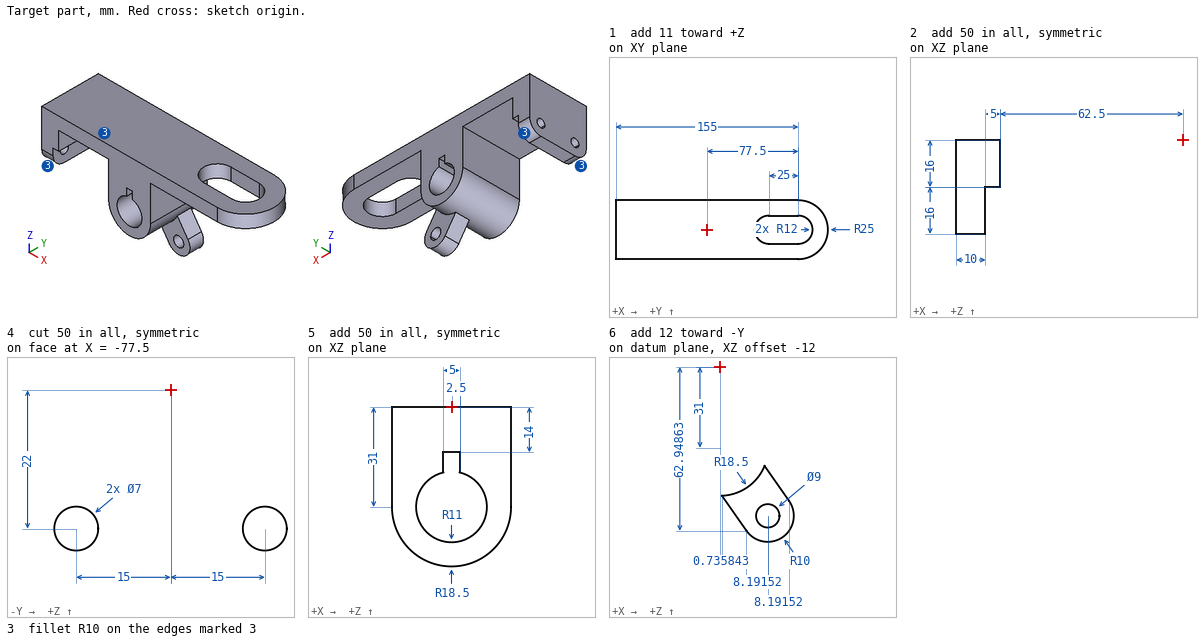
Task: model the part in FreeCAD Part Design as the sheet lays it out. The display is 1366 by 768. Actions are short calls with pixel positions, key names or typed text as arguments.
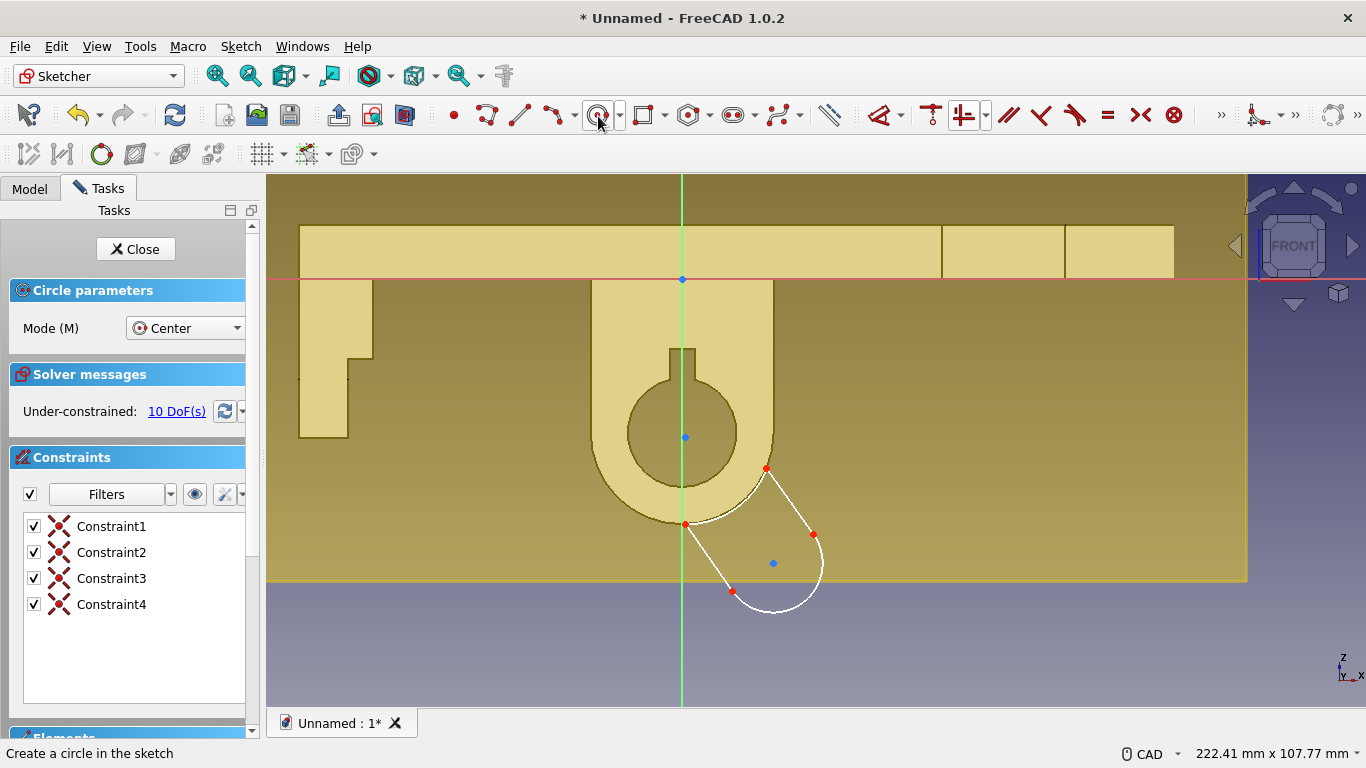
click(773, 562)
click(789, 547)
key(Escape)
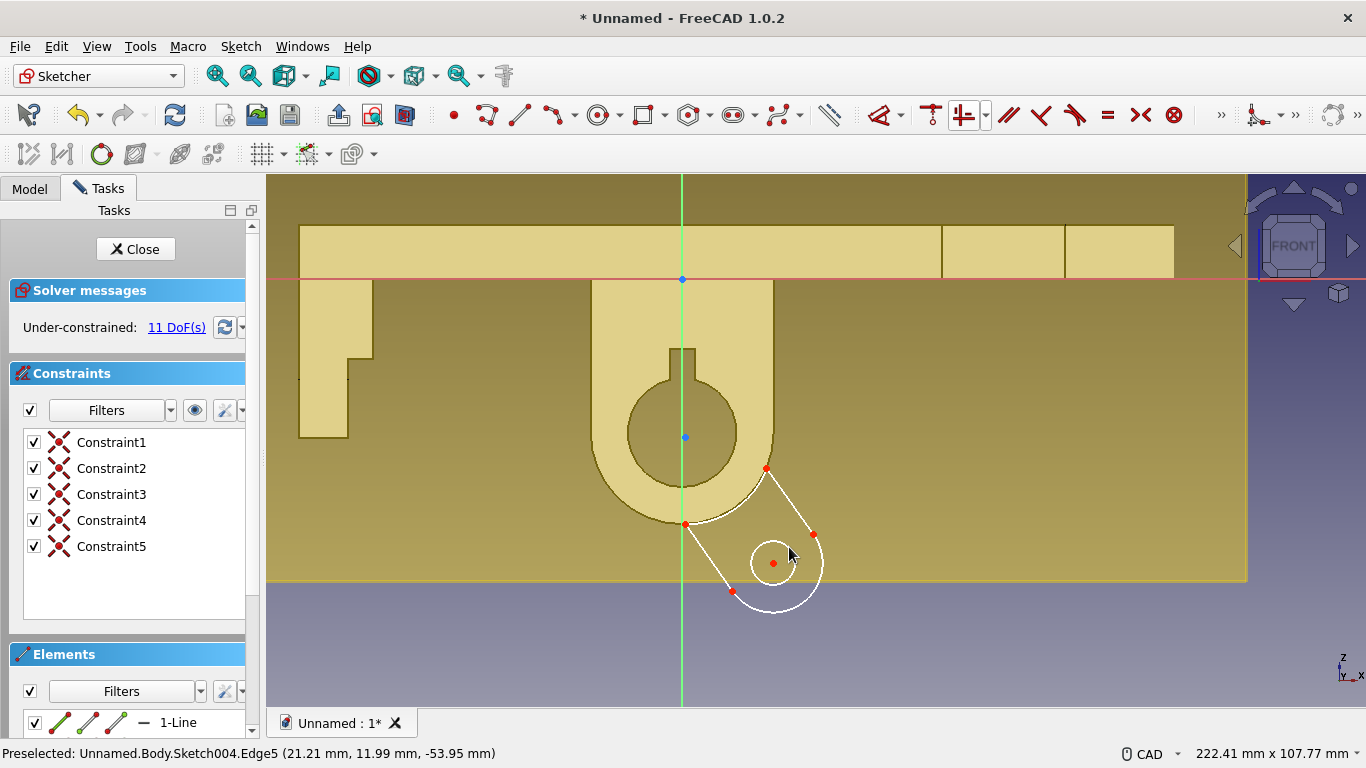
click(781, 489)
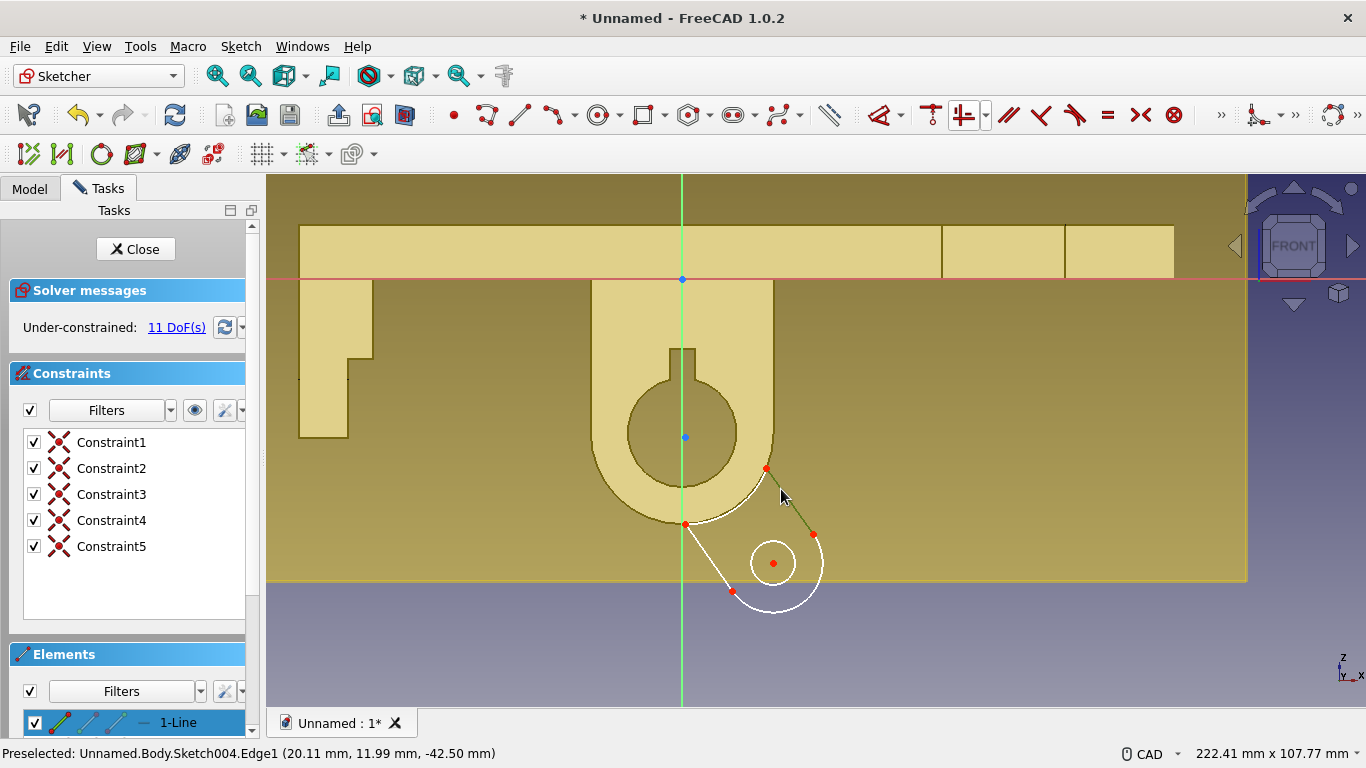
click(772, 613)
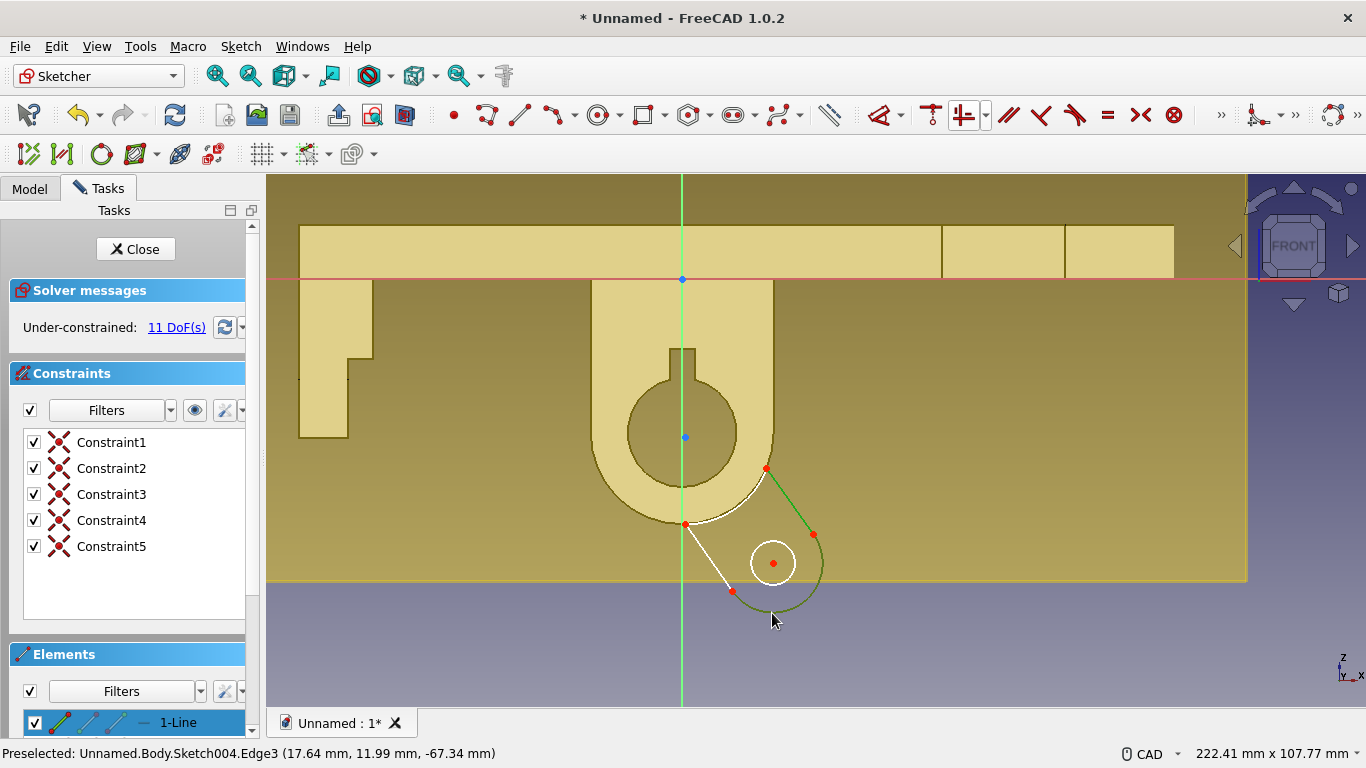
click(1075, 116)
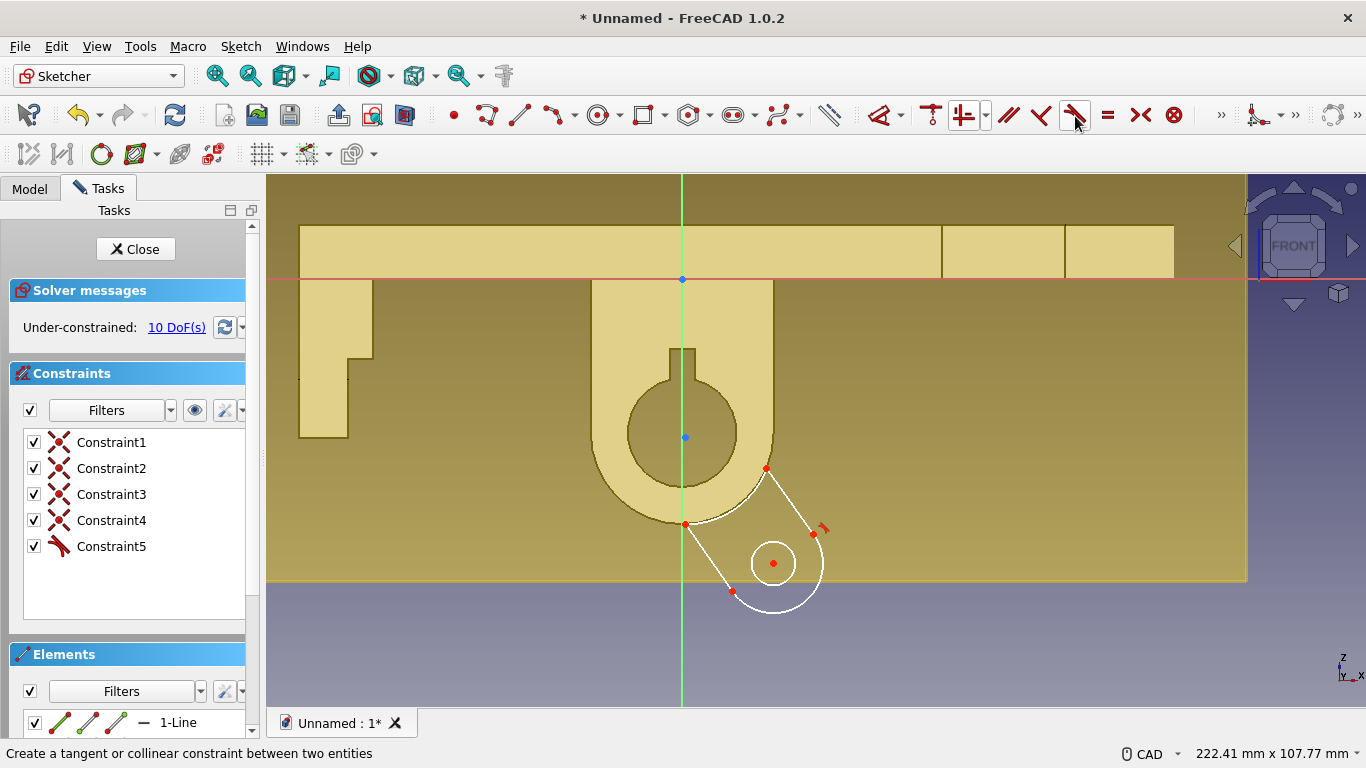
click(719, 572)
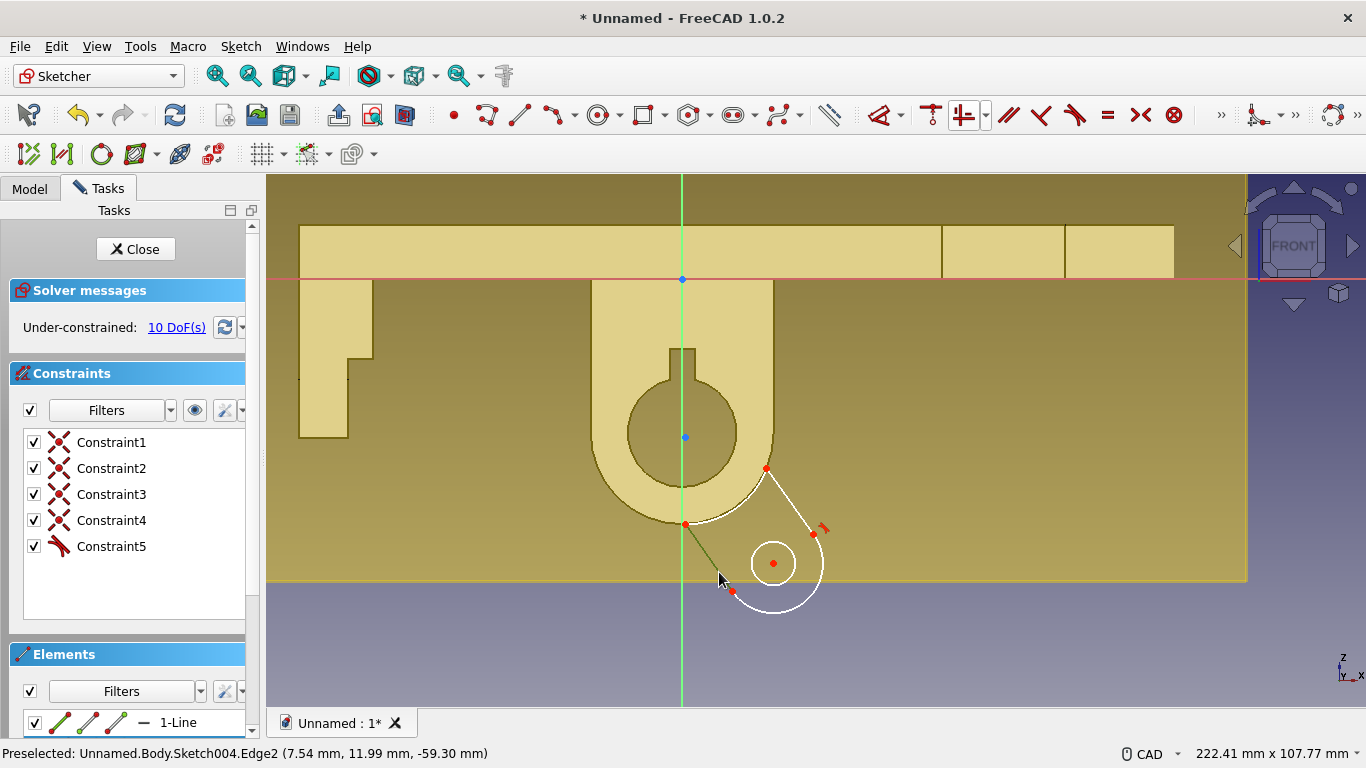
click(773, 613)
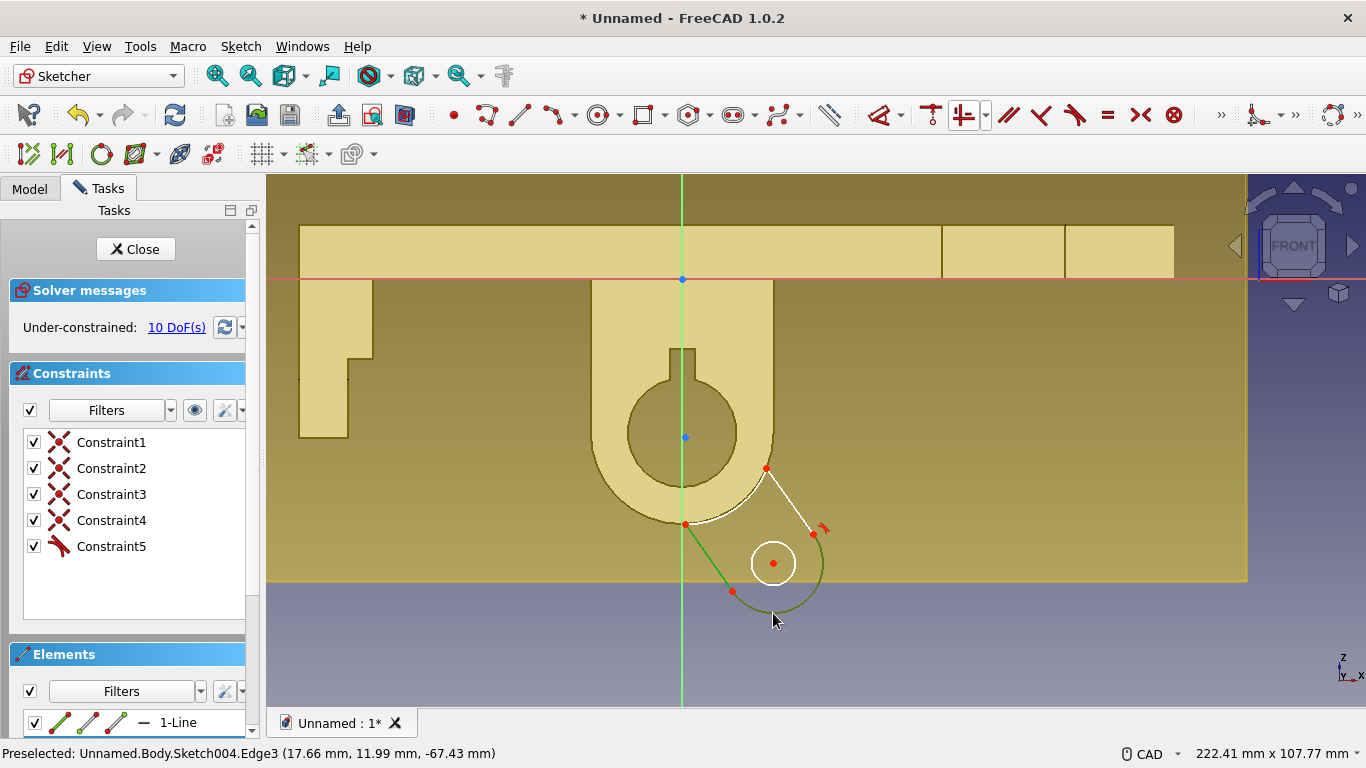
click(1075, 116)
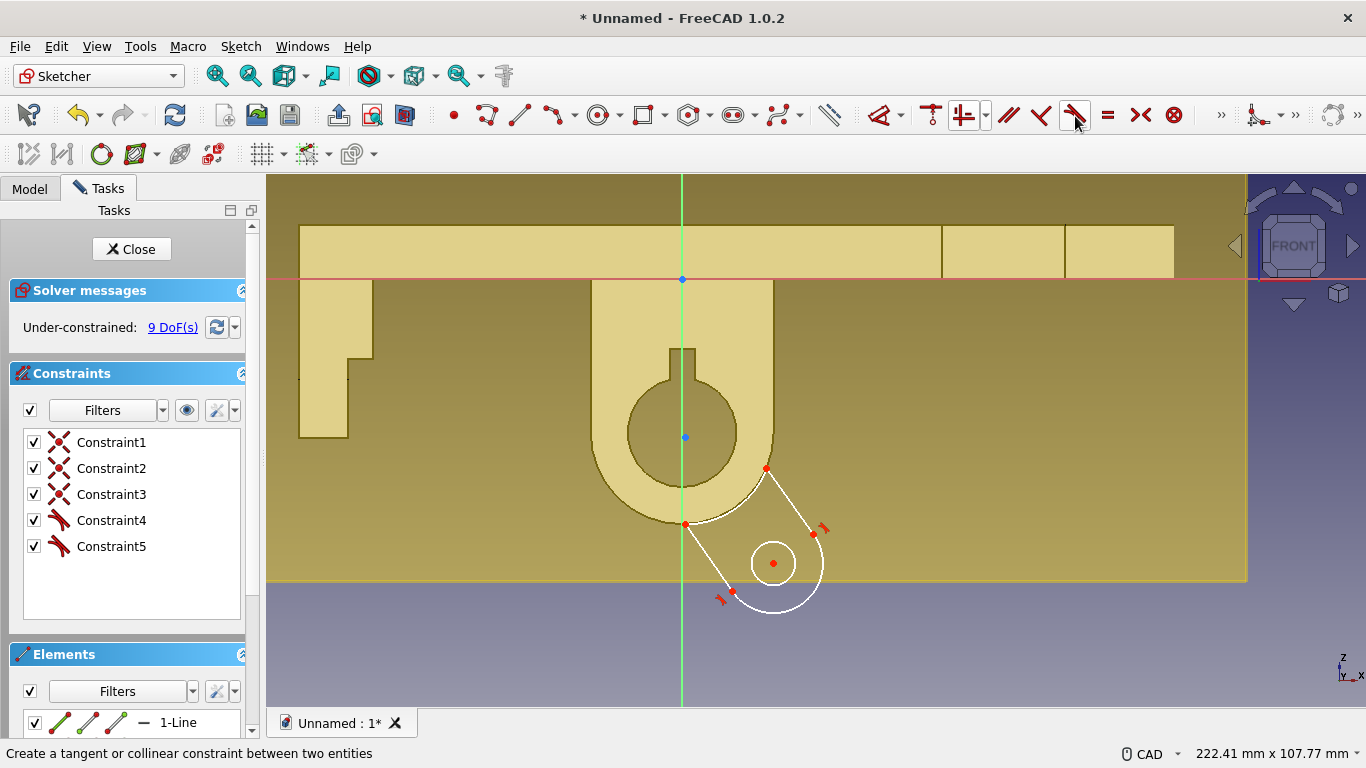
click(686, 437)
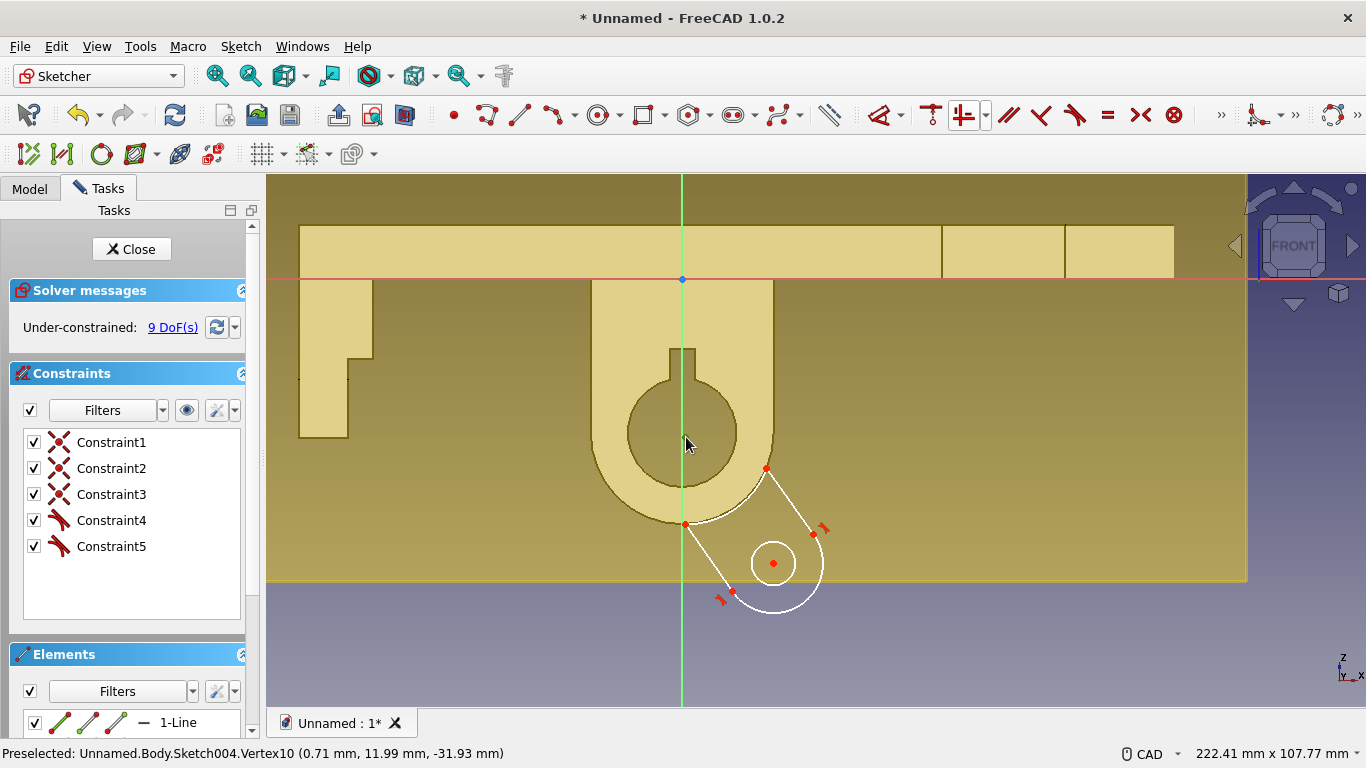
click(682, 645)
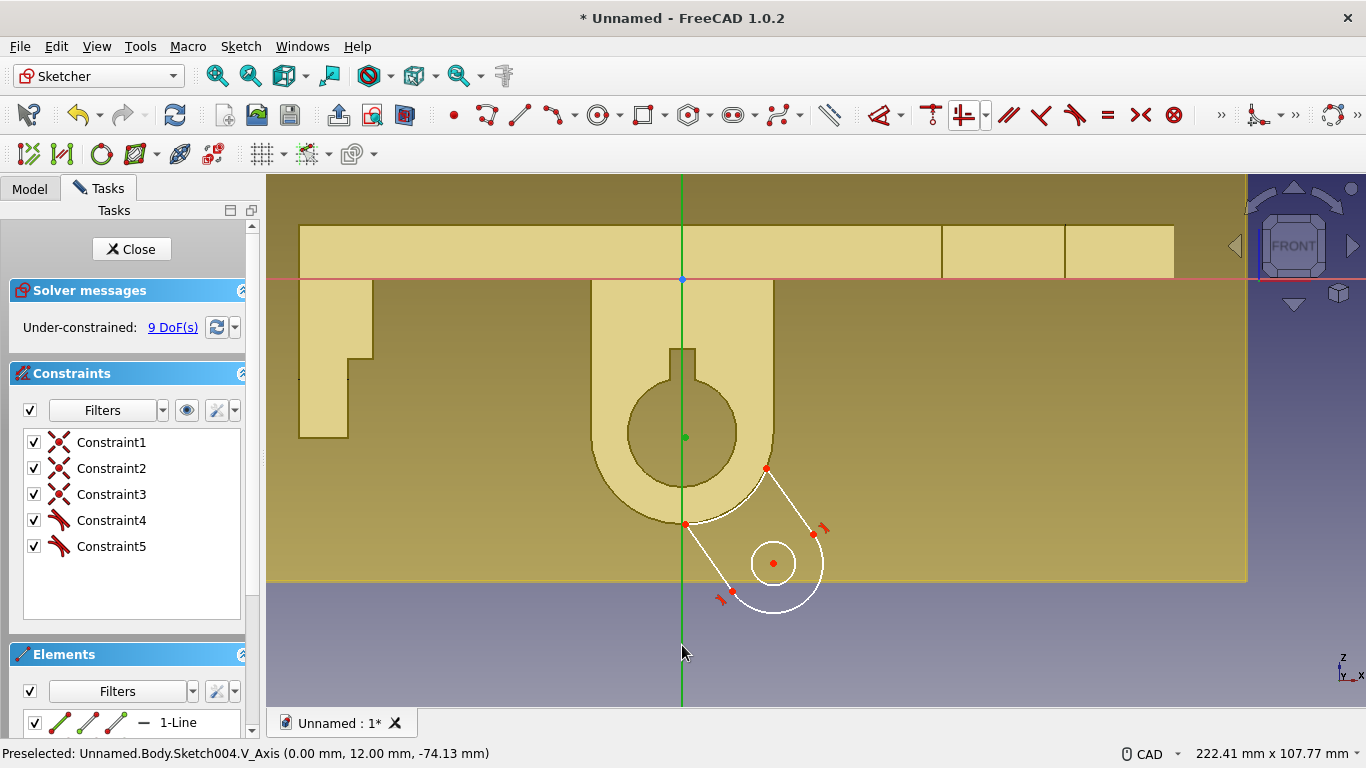
click(931, 116)